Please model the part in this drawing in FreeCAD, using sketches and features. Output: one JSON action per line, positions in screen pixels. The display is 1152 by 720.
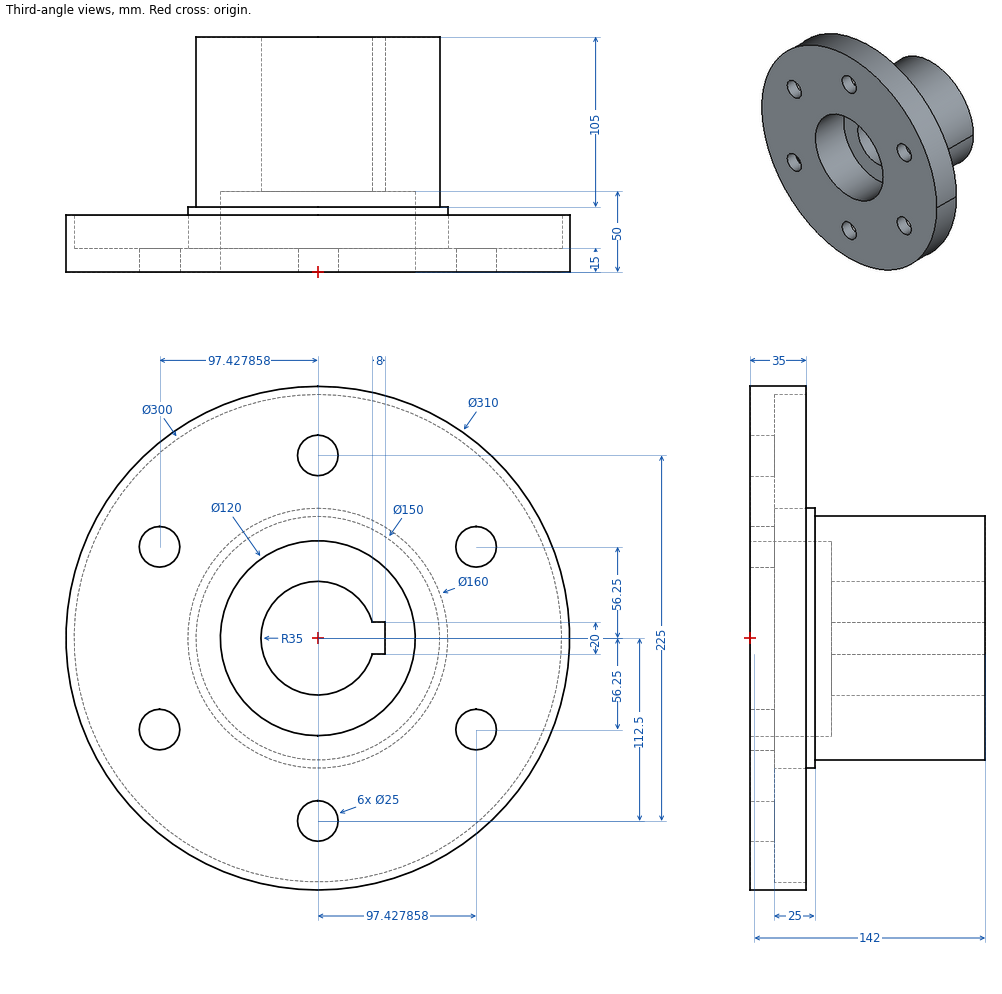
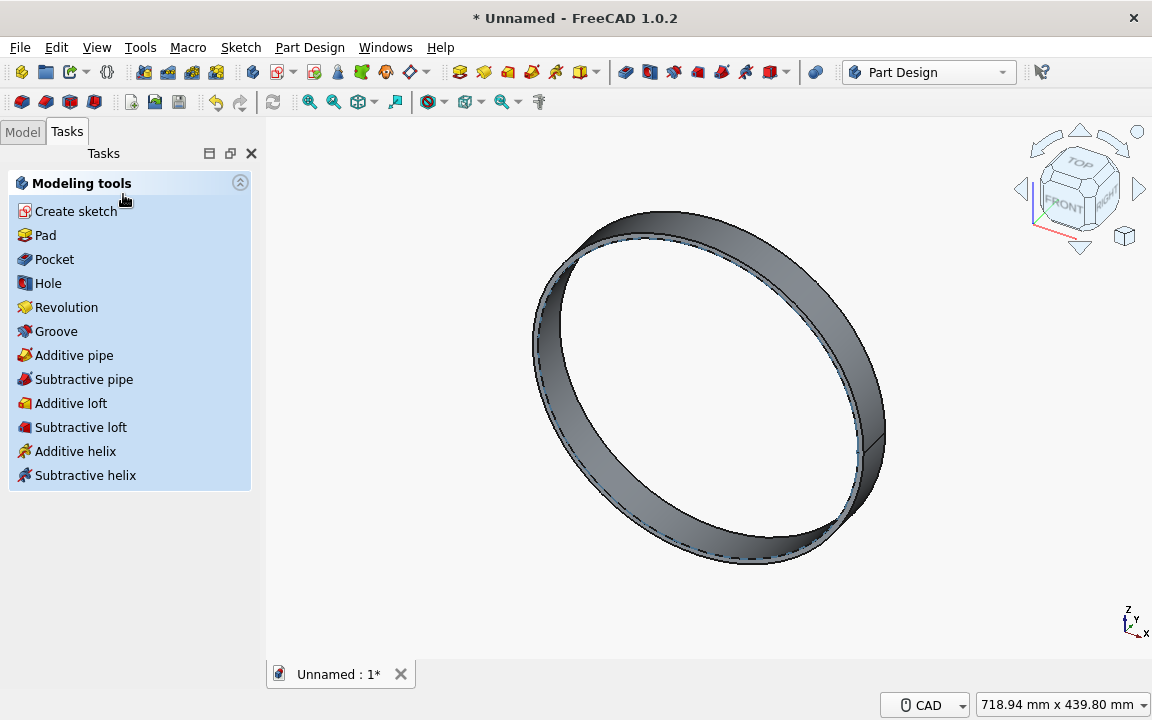
{"action": "left_click", "coordinate": [460, 72]}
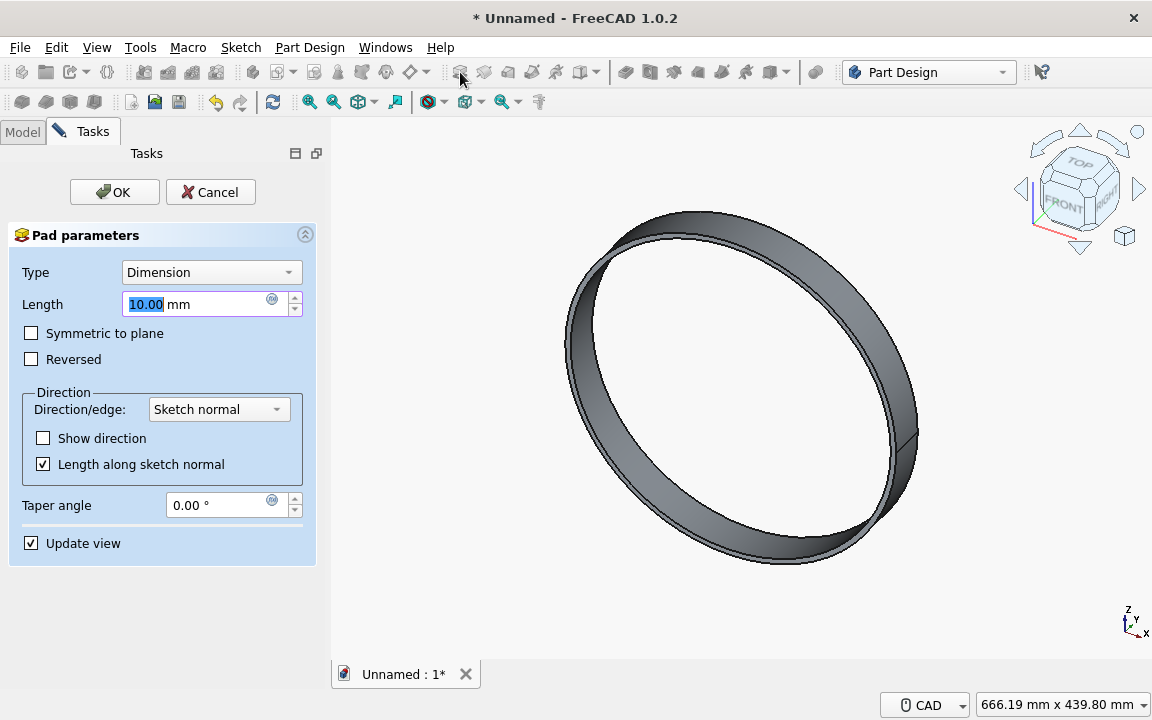
{"action": "type", "text": "15"}
{"action": "key", "text": "Tab"}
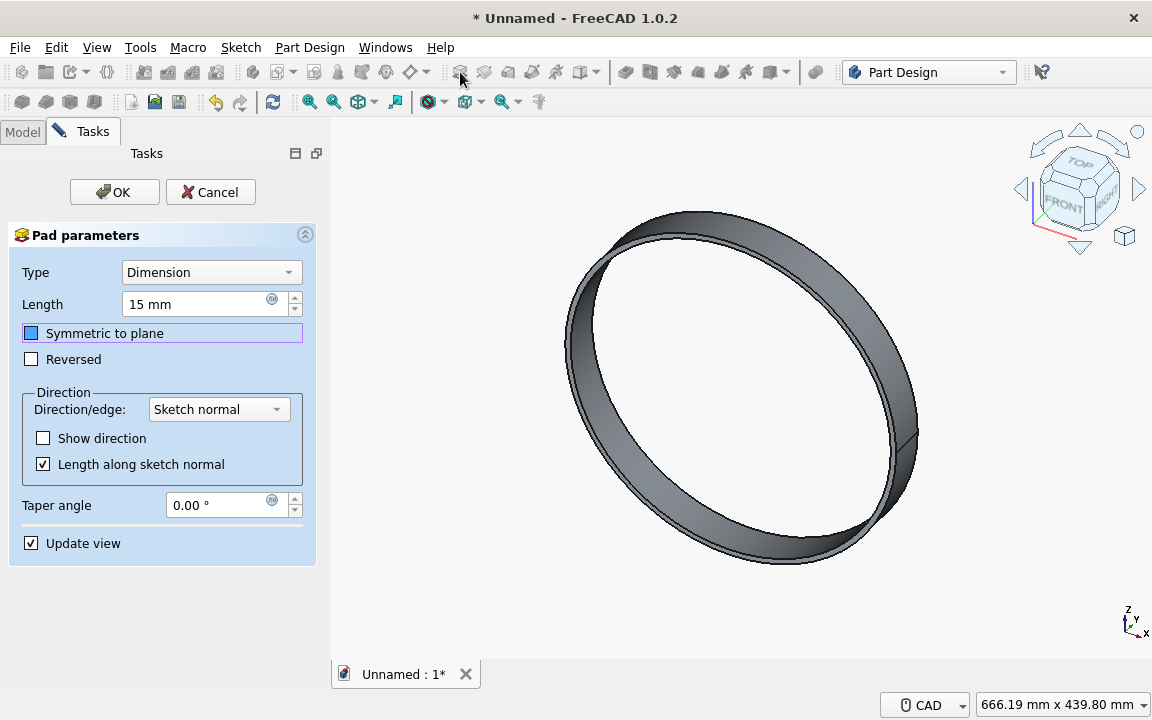
{"action": "left_click", "coordinate": [30, 359]}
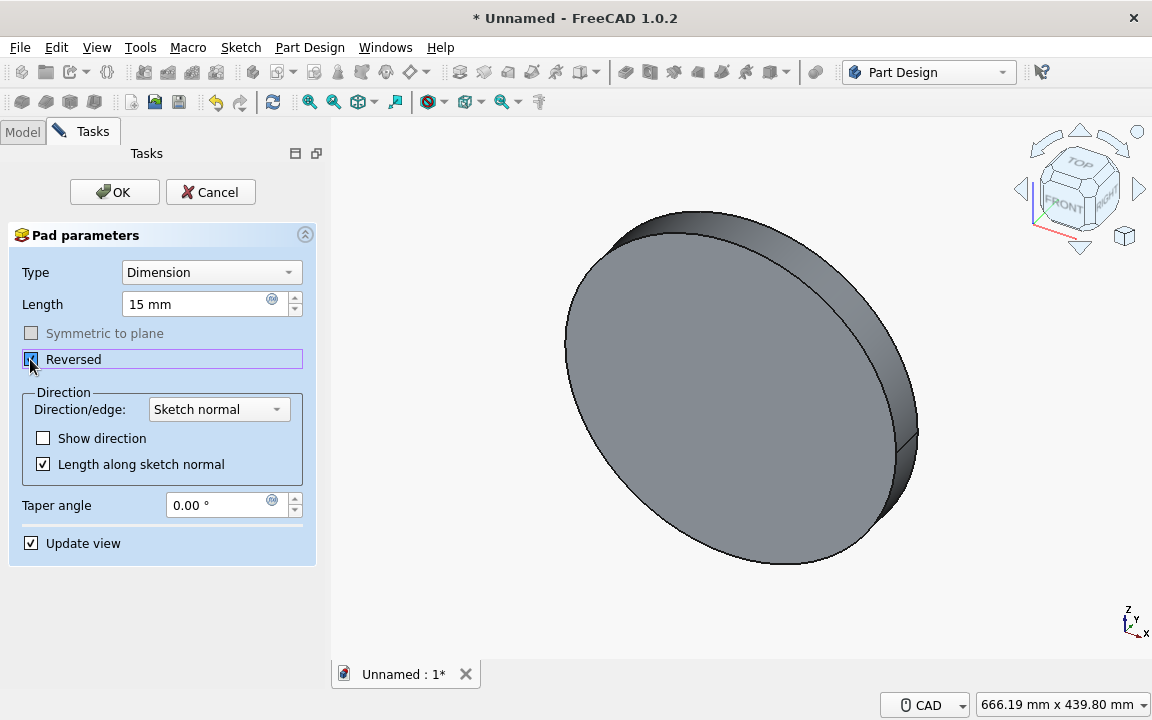
{"action": "left_click", "coordinate": [115, 192]}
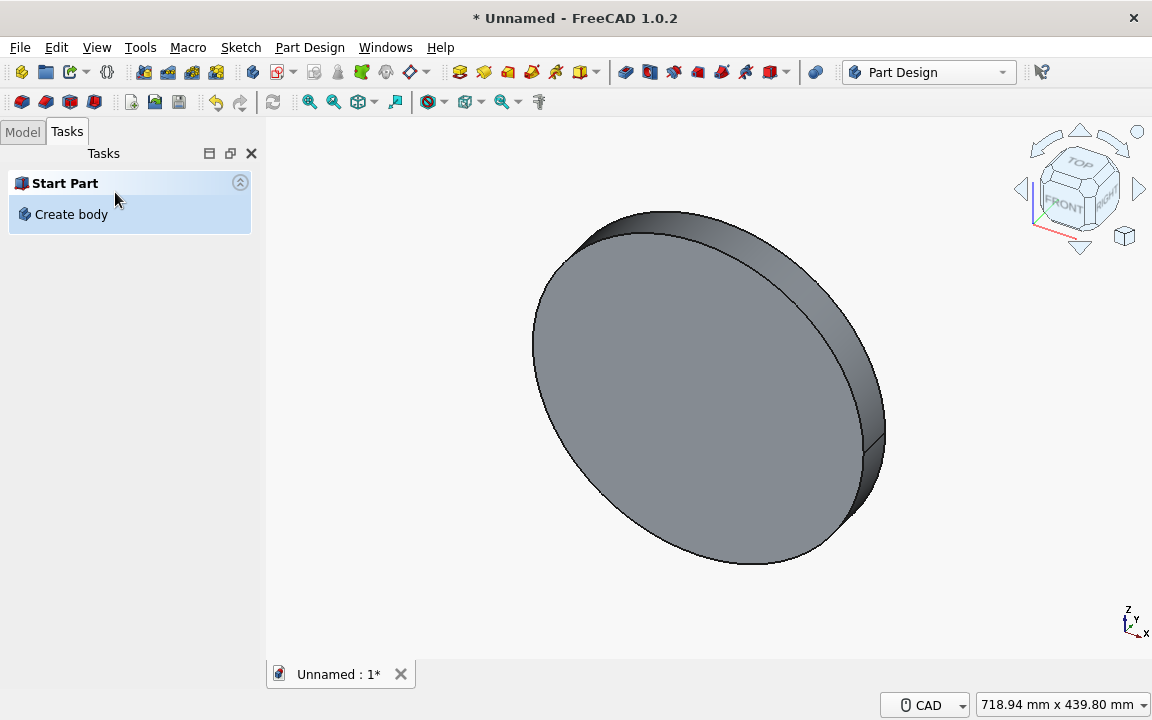
{"action": "key", "text": "4"}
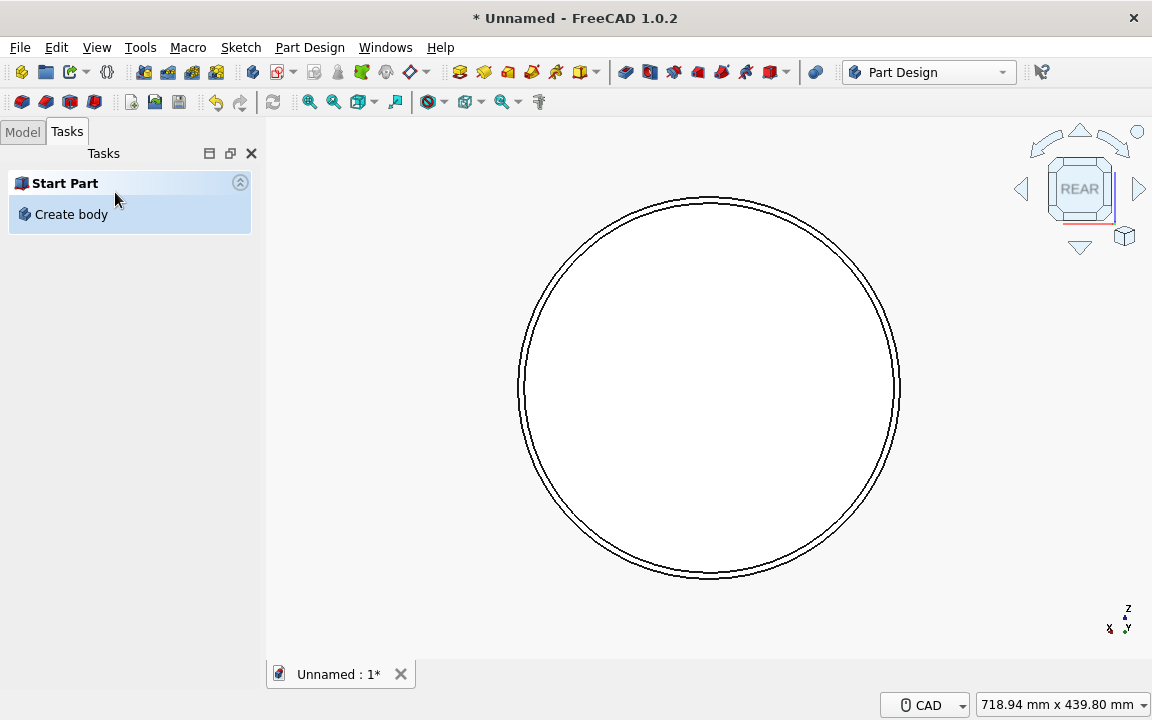
{"action": "left_click", "coordinate": [709, 387]}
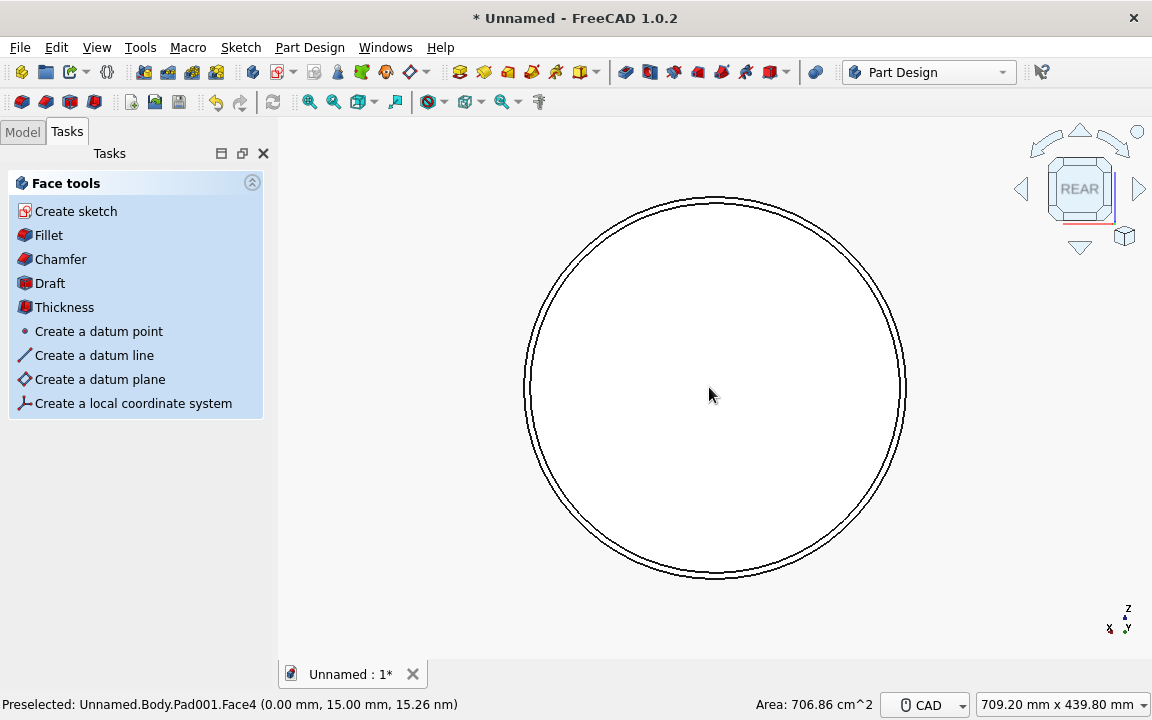
{"action": "left_click", "coordinate": [278, 72]}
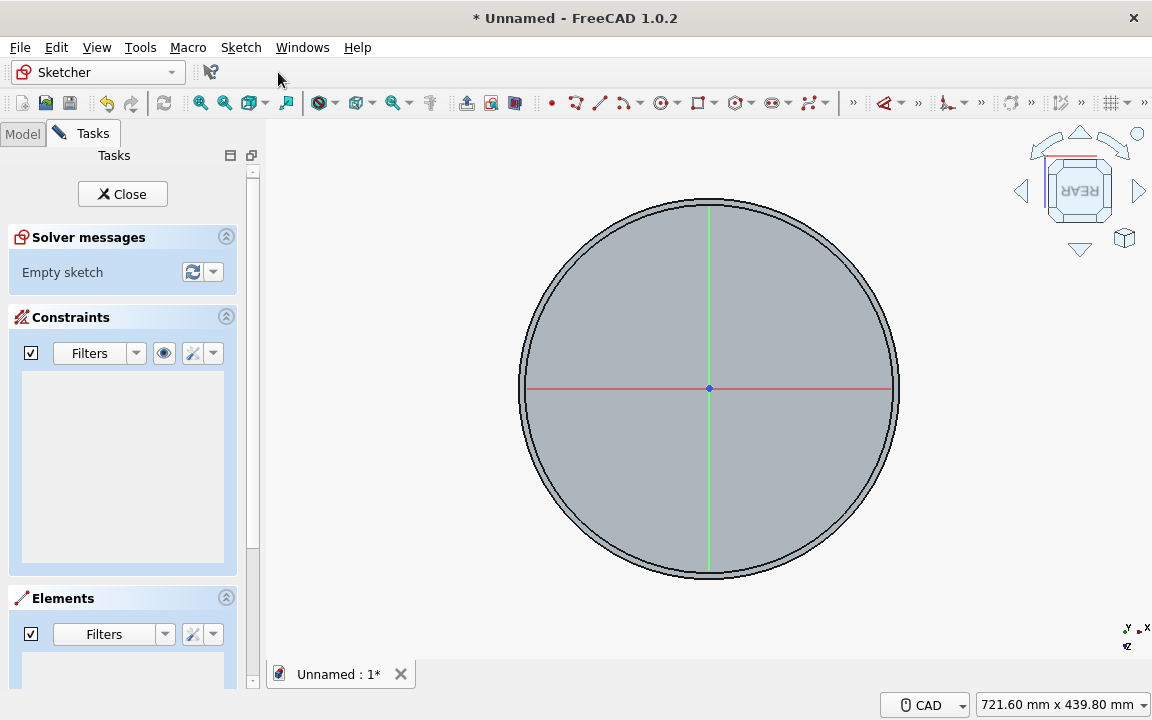
{"action": "left_click", "coordinate": [516, 104]}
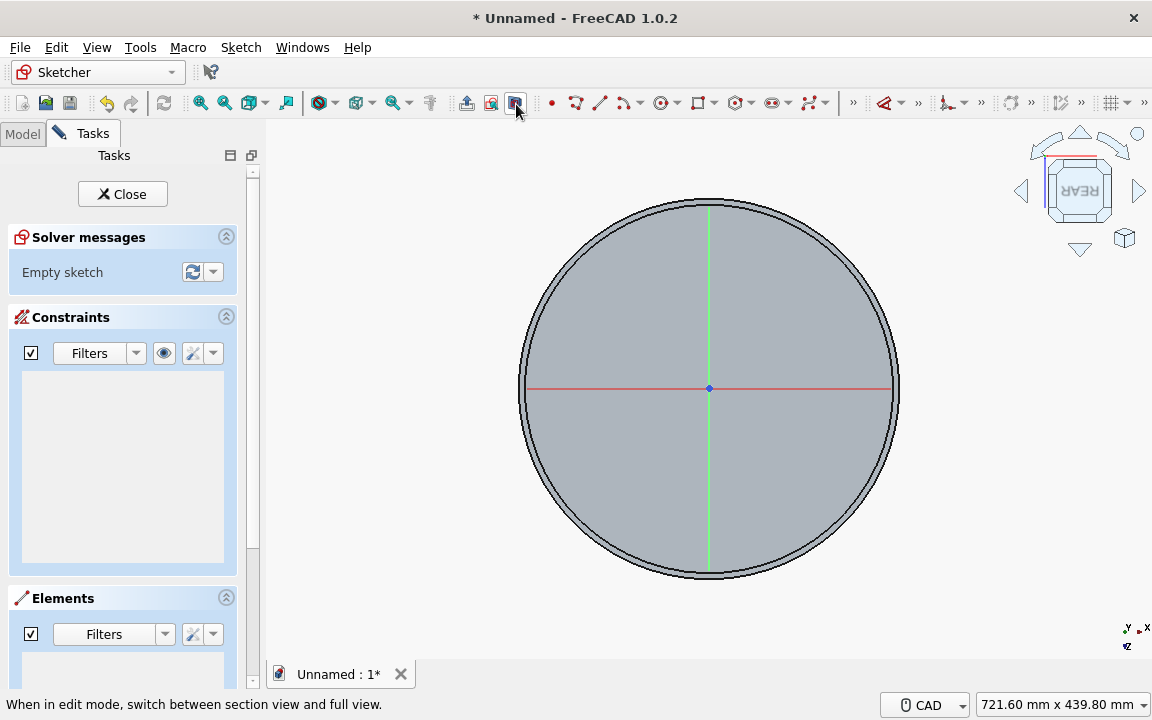
{"action": "left_click", "coordinate": [662, 104]}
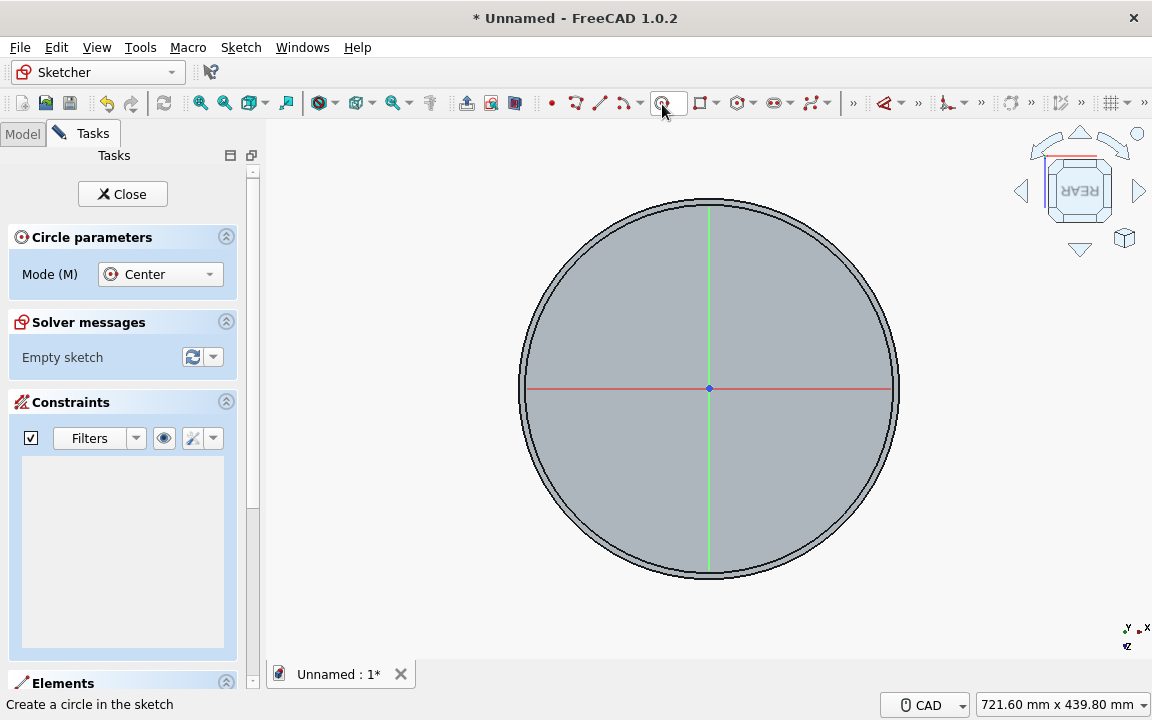
{"action": "scroll", "coordinate": [709, 251], "scroll_direction": "up", "scroll_amount": 2}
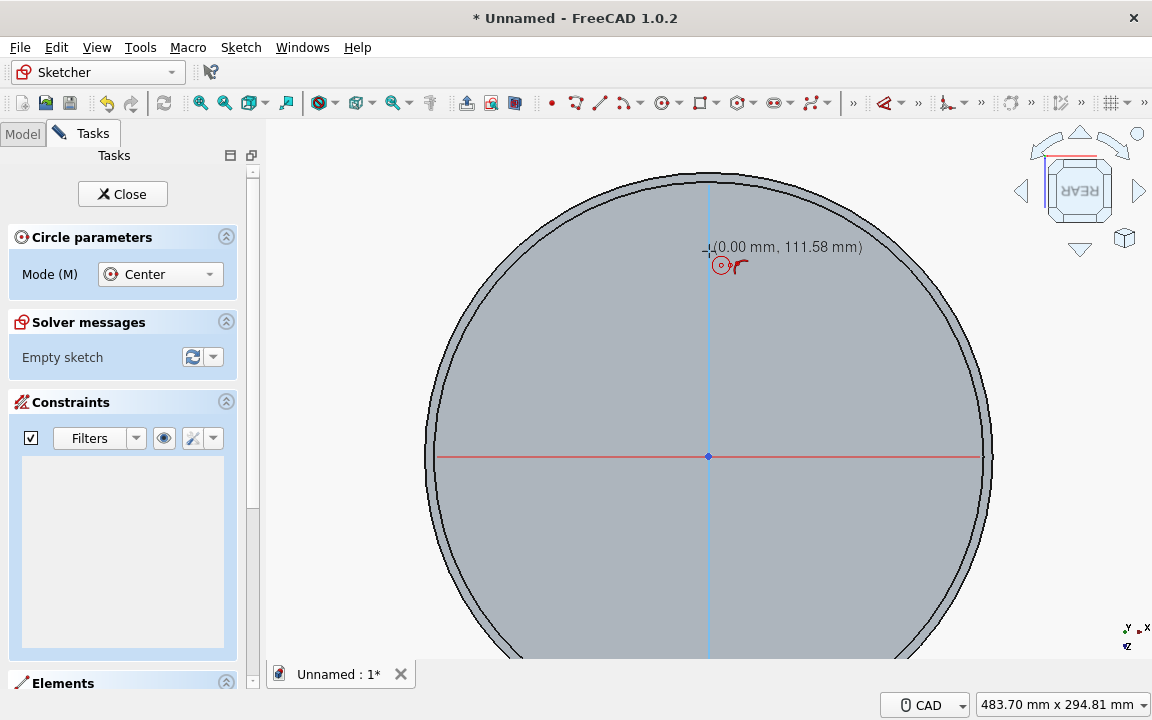
{"action": "left_click", "coordinate": [709, 251]}
{"action": "mouse_move", "coordinate": [725, 234]}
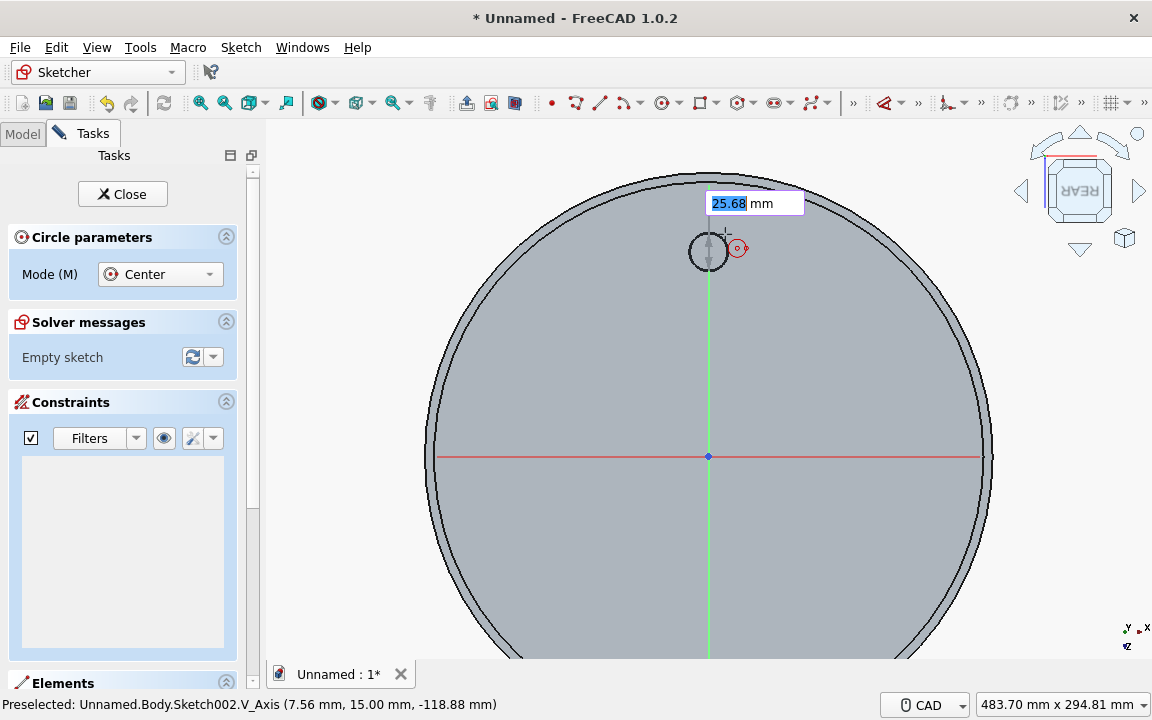
{"action": "type", "text": "25"}
{"action": "key", "text": "Return"}